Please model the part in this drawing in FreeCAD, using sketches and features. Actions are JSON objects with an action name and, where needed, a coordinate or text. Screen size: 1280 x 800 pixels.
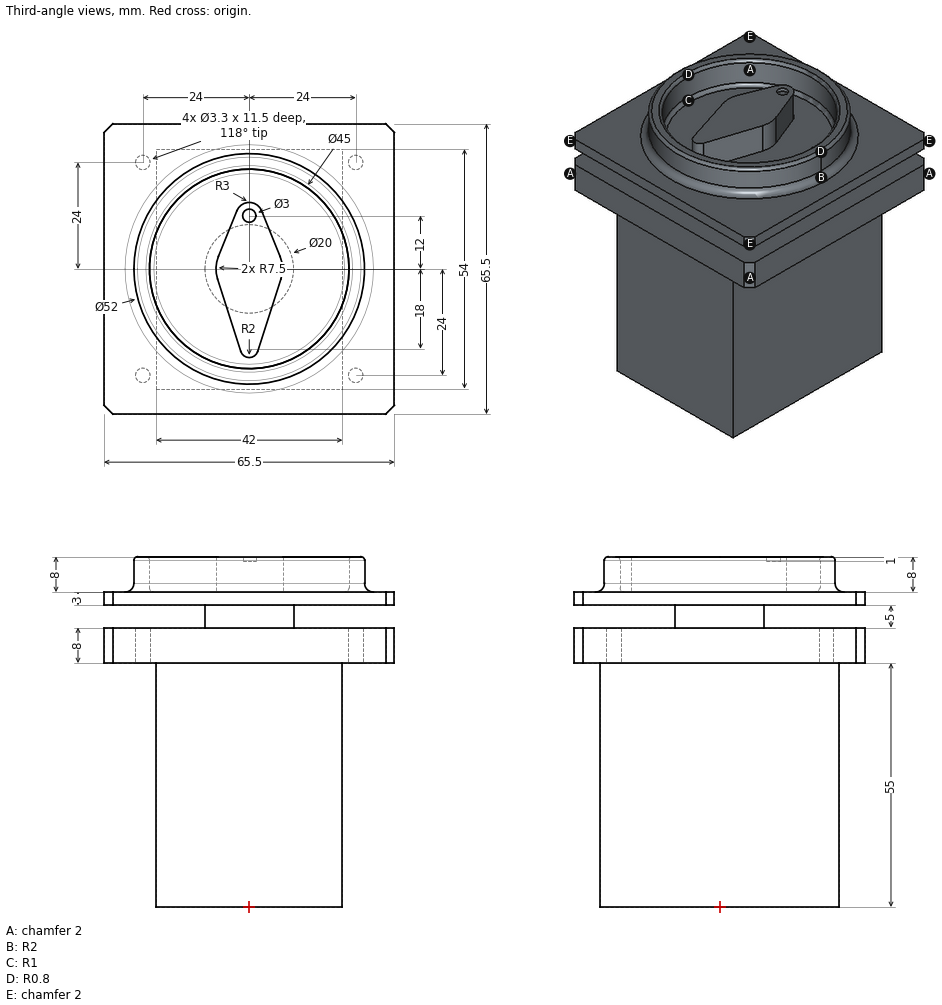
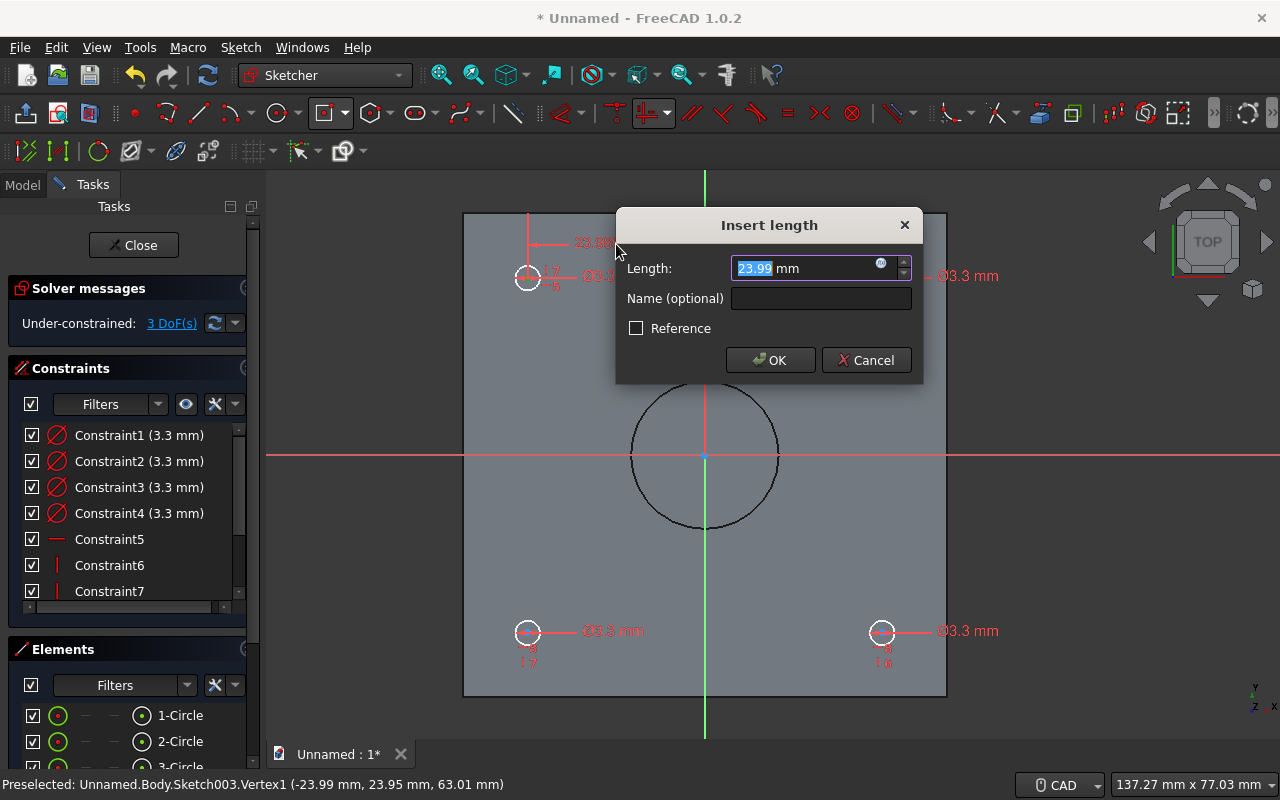
{"action": "type", "text": "24"}
{"action": "key", "text": "Return"}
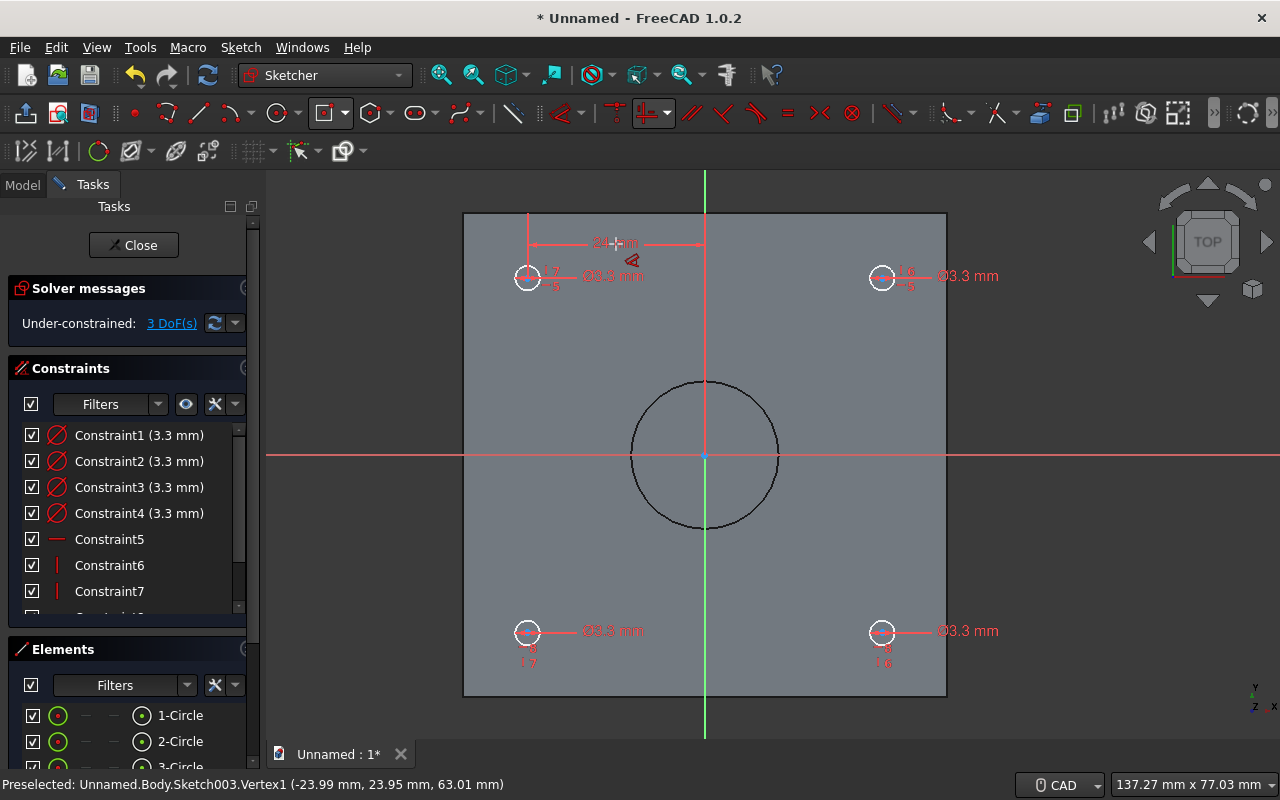
{"action": "left_click", "coordinate": [528, 278]}
{"action": "left_click", "coordinate": [494, 367]}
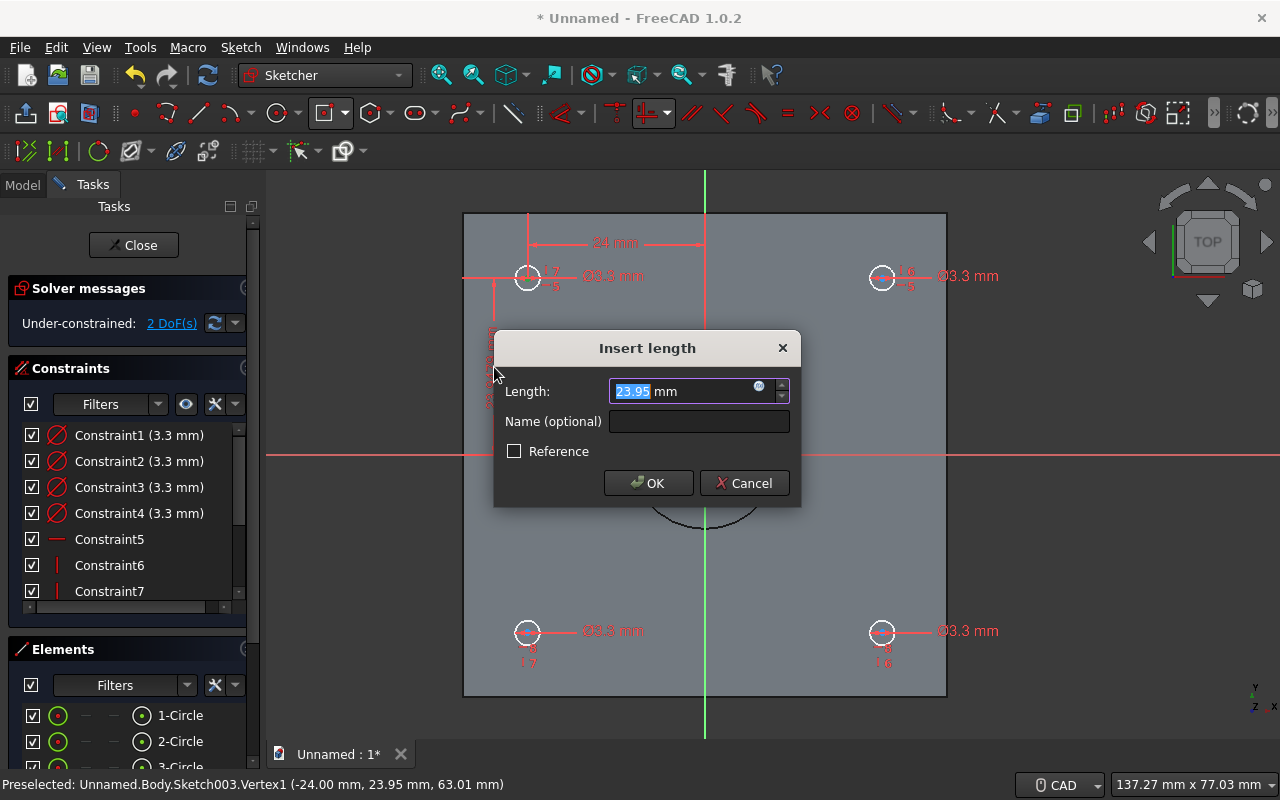
{"action": "type", "text": "24"}
{"action": "key", "text": "Return"}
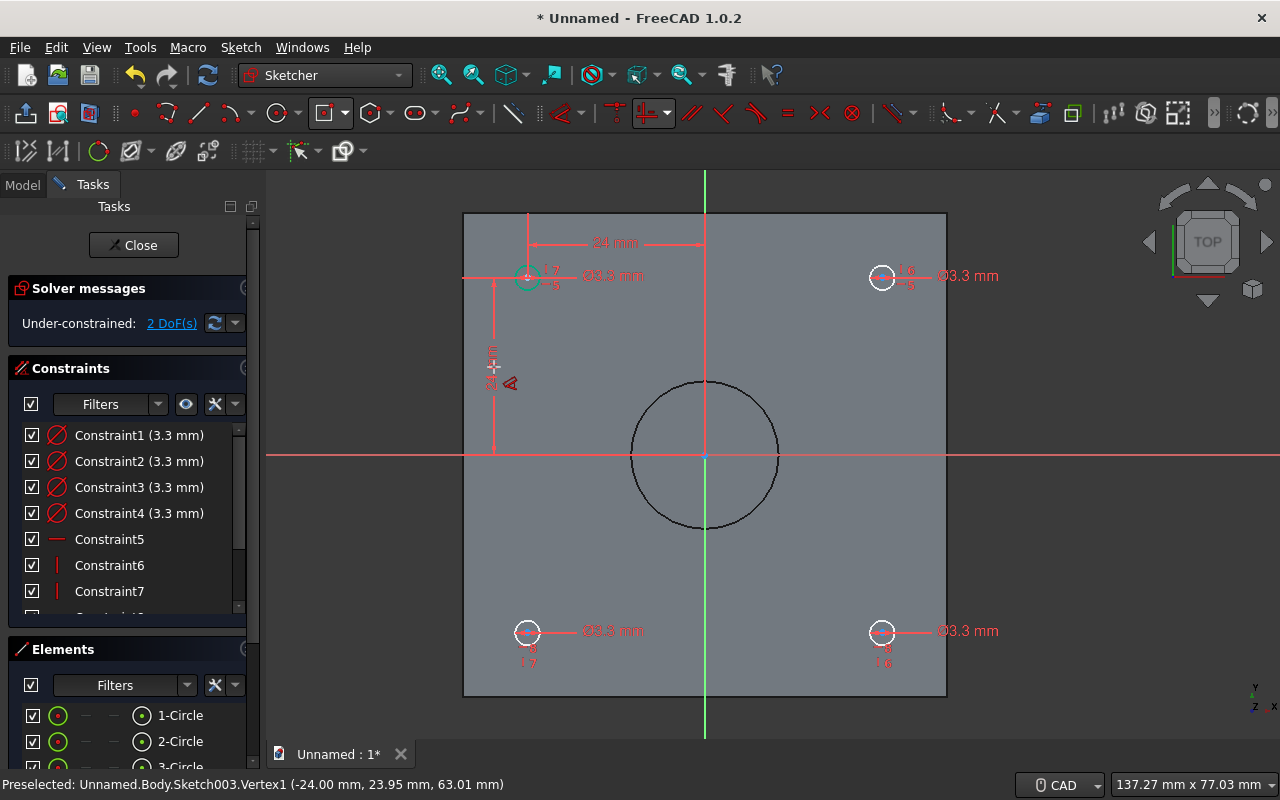
{"action": "left_click", "coordinate": [882, 278]}
{"action": "left_click", "coordinate": [794, 244]}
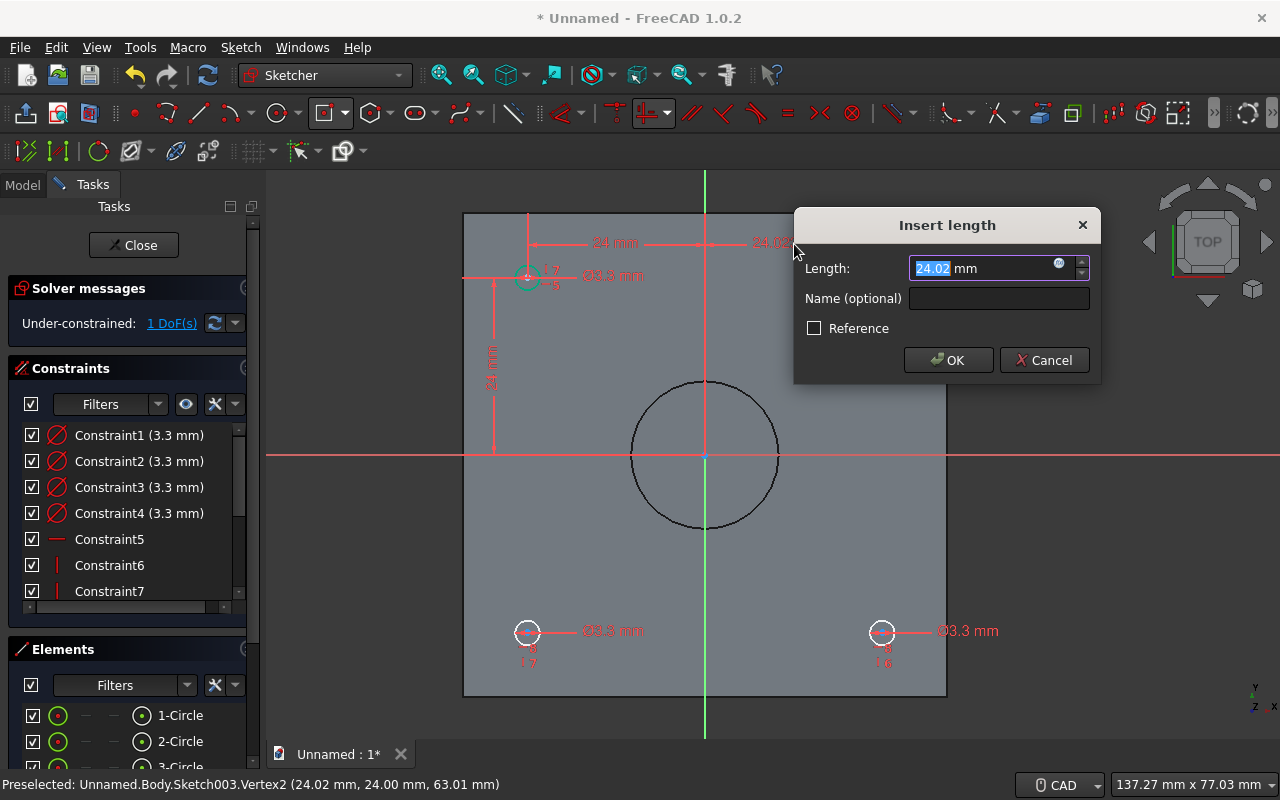
{"action": "type", "text": "24"}
{"action": "key", "text": "Return"}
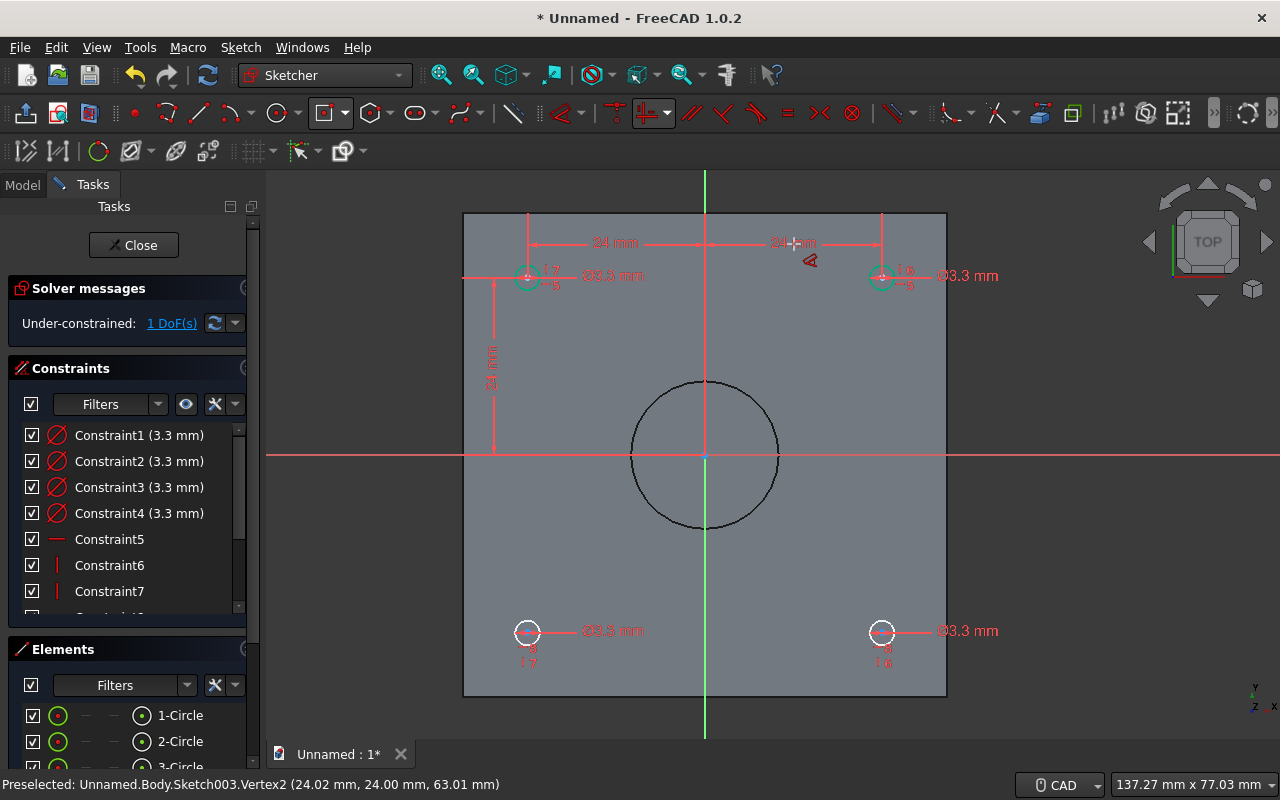
{"action": "left_click", "coordinate": [882, 633]}
{"action": "left_click", "coordinate": [916, 544]}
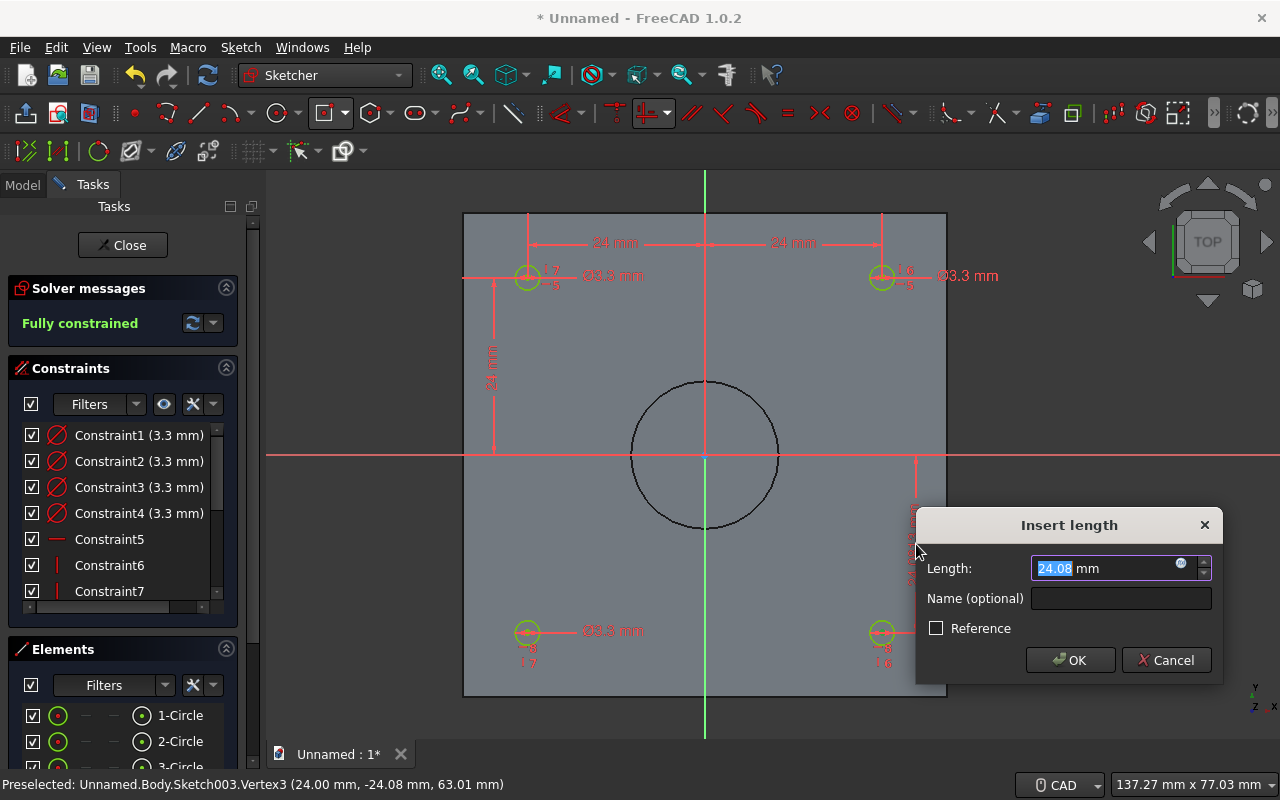
{"action": "type", "text": "24"}
{"action": "key", "text": "Return"}
{"action": "key", "text": "Escape"}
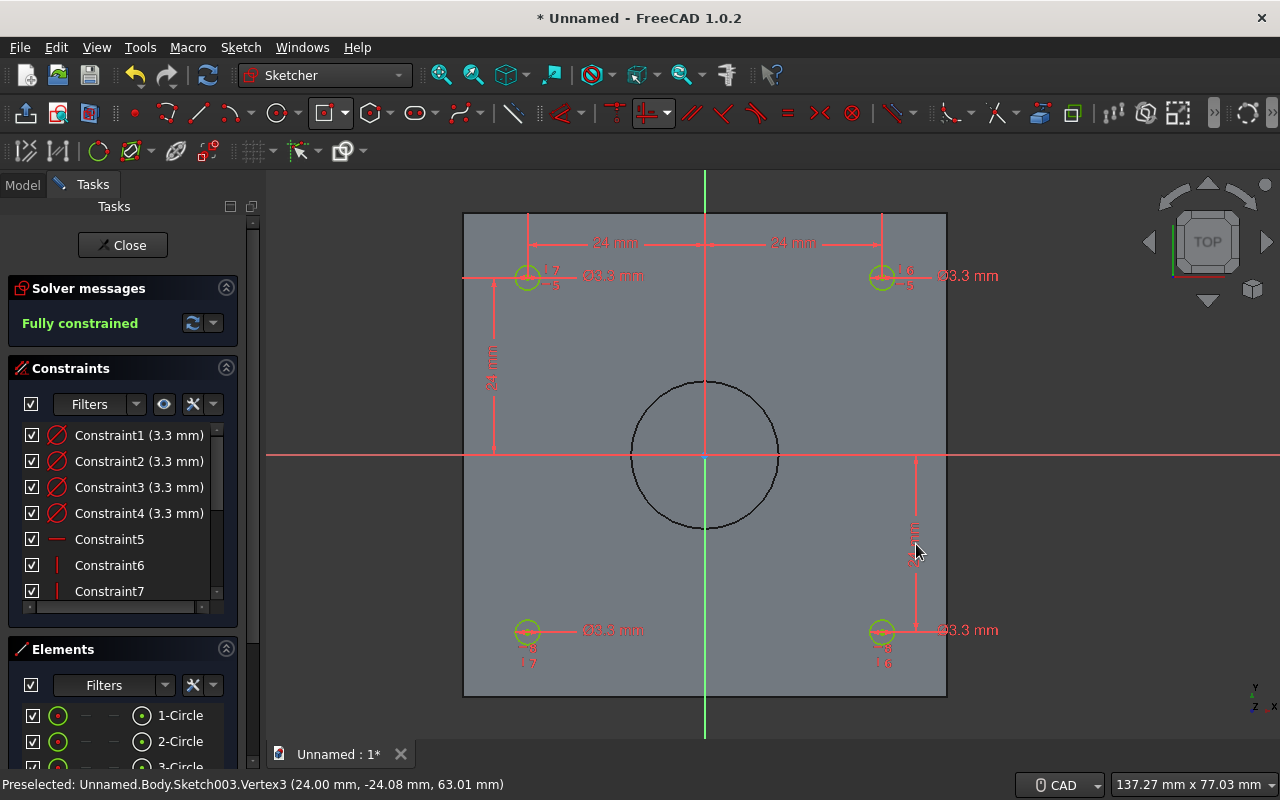
{"action": "left_click", "coordinate": [123, 245]}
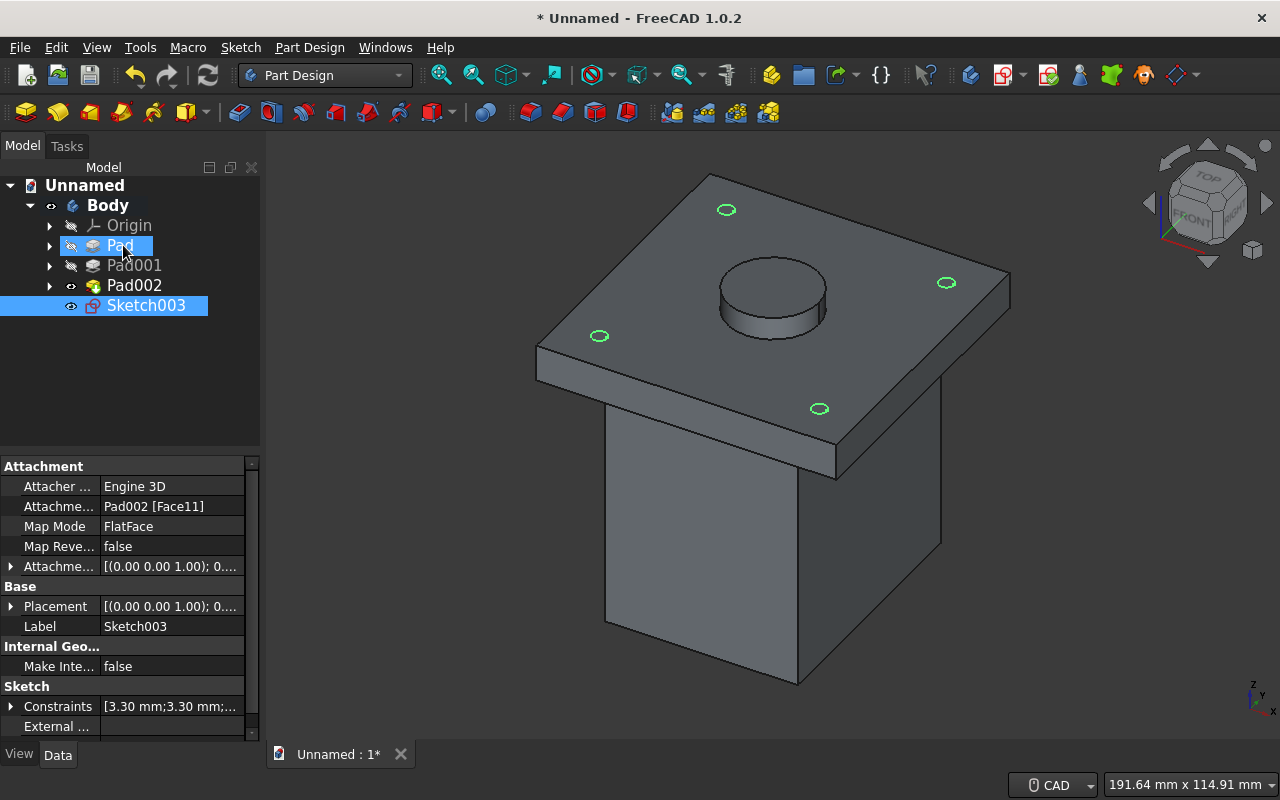
{"action": "left_click", "coordinate": [272, 112]}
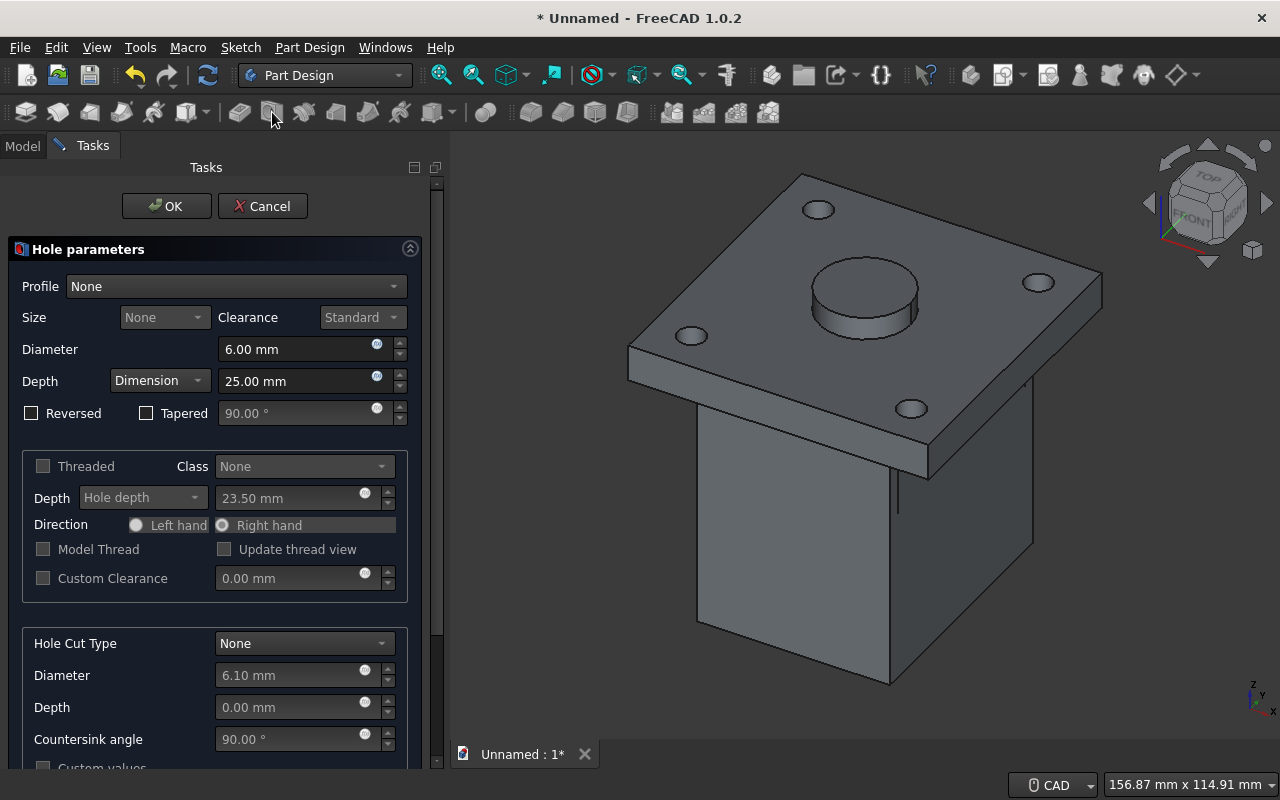
{"action": "triple_click", "coordinate": [305, 349]}